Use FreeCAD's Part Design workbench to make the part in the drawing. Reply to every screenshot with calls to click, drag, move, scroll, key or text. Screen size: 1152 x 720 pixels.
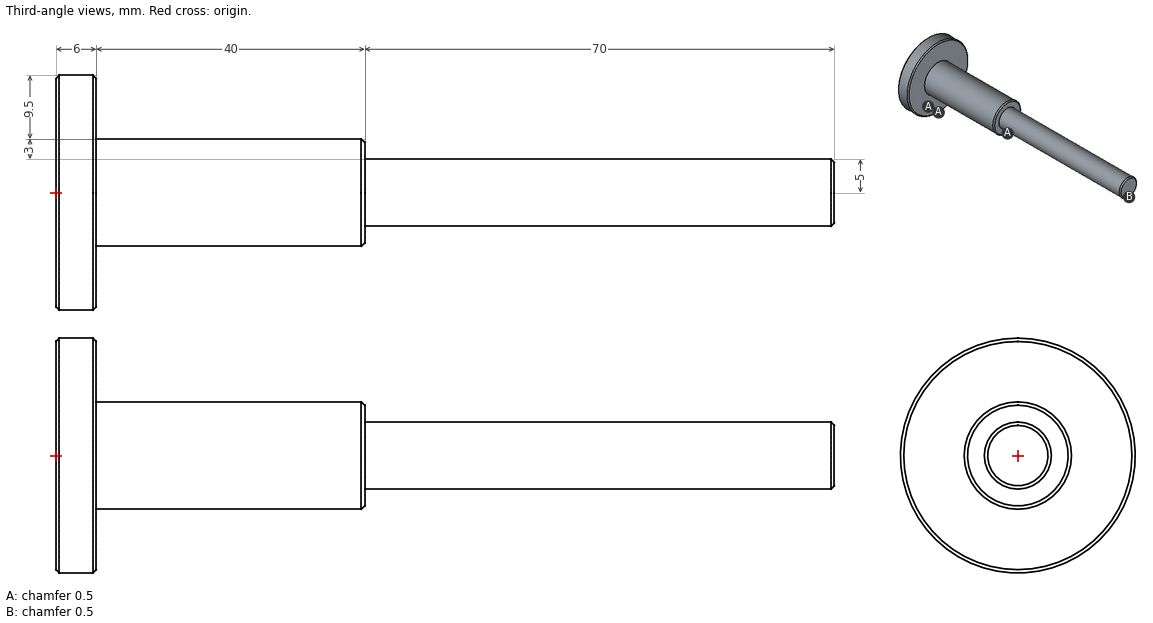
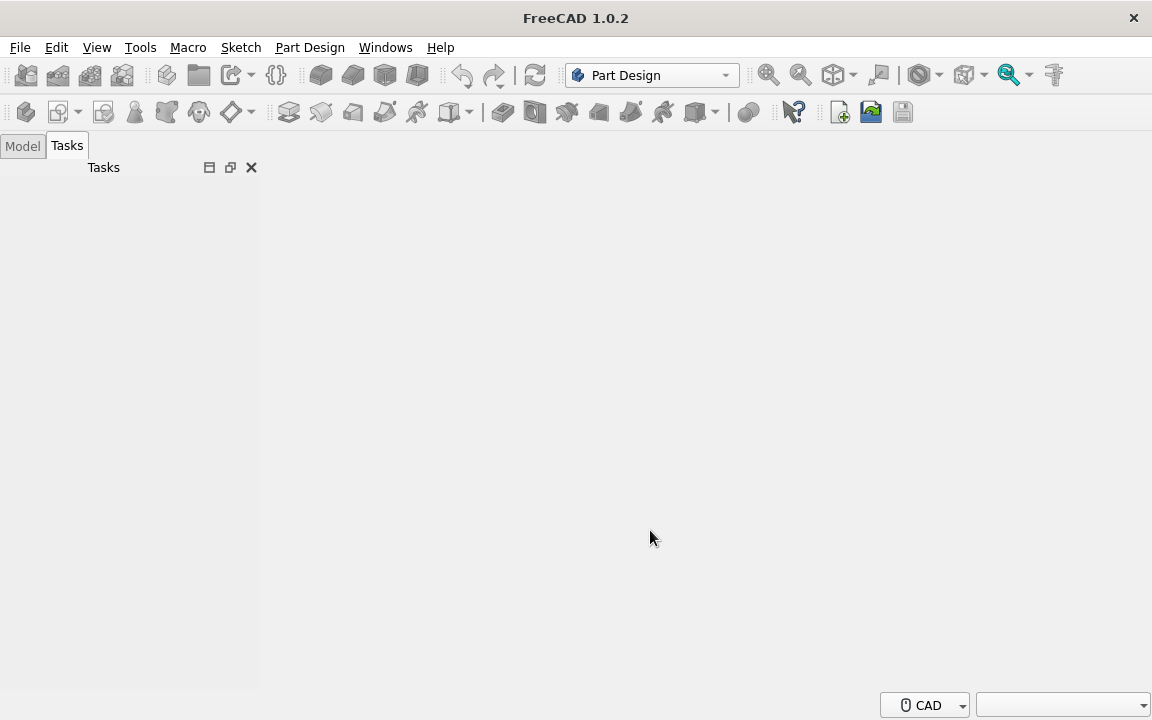
click(840, 112)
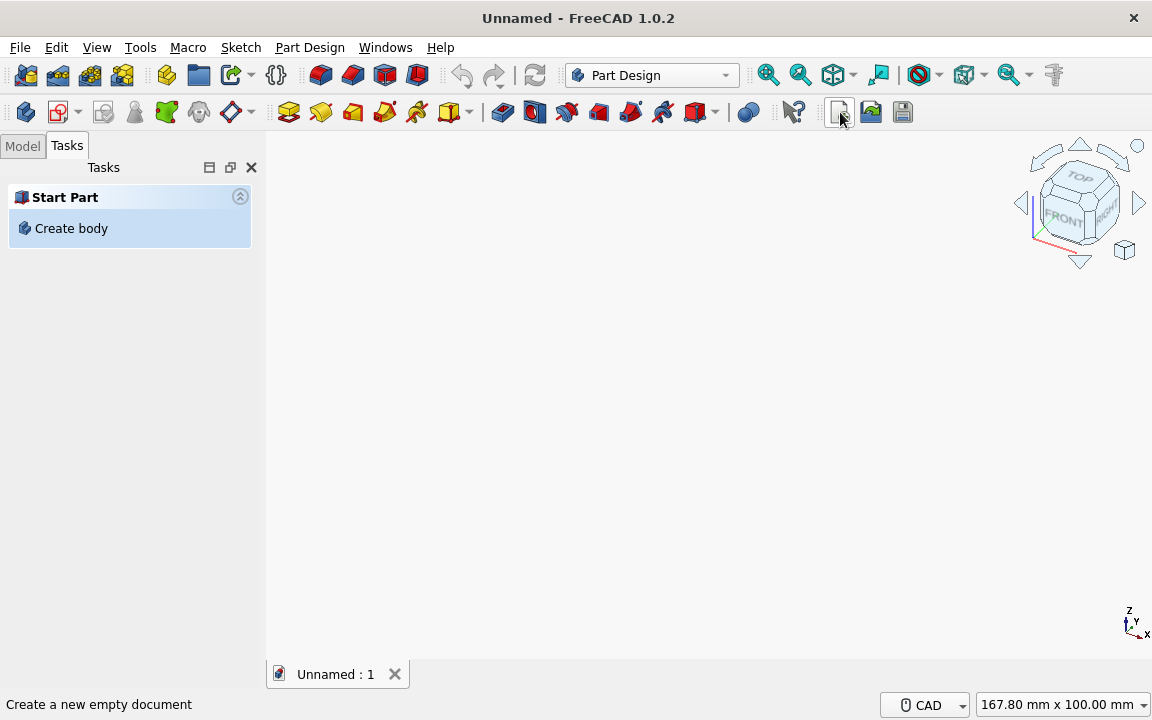
click(58, 112)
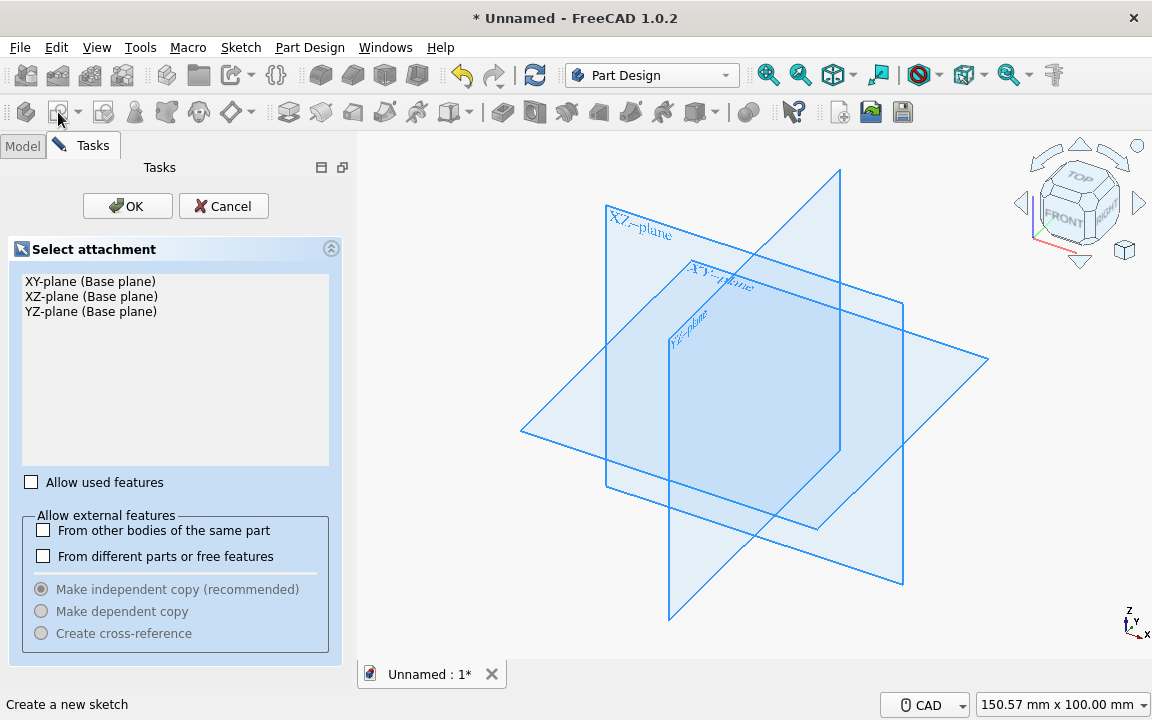
click(82, 282)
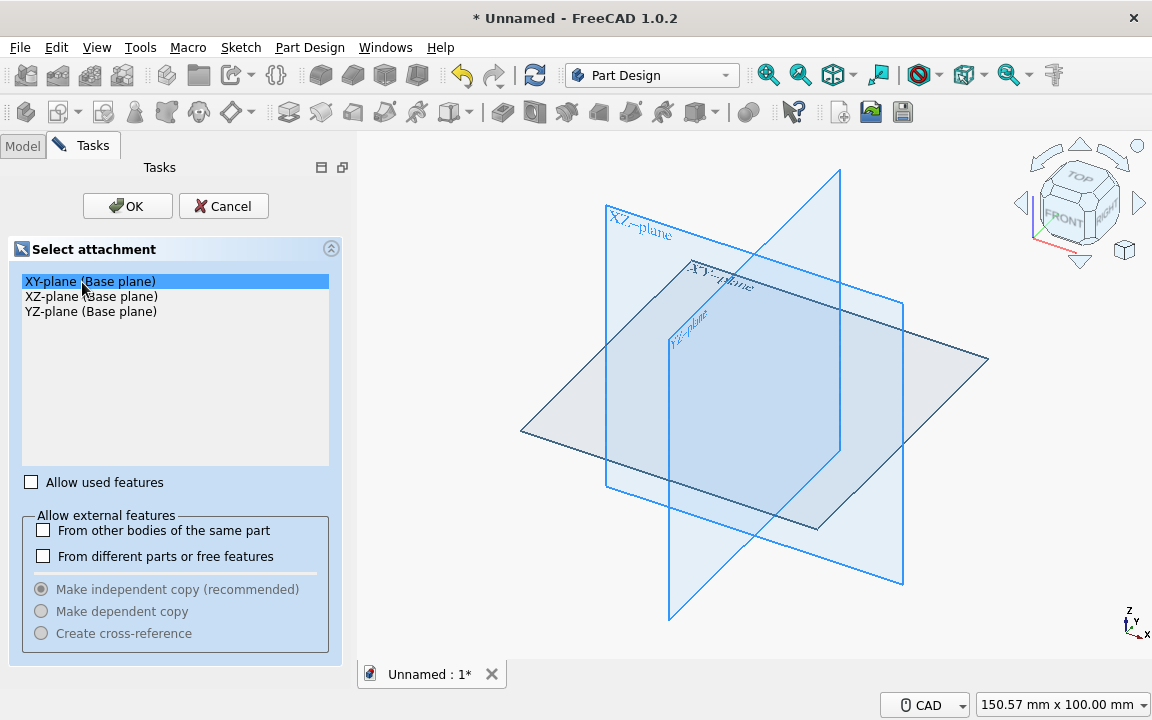
click(128, 206)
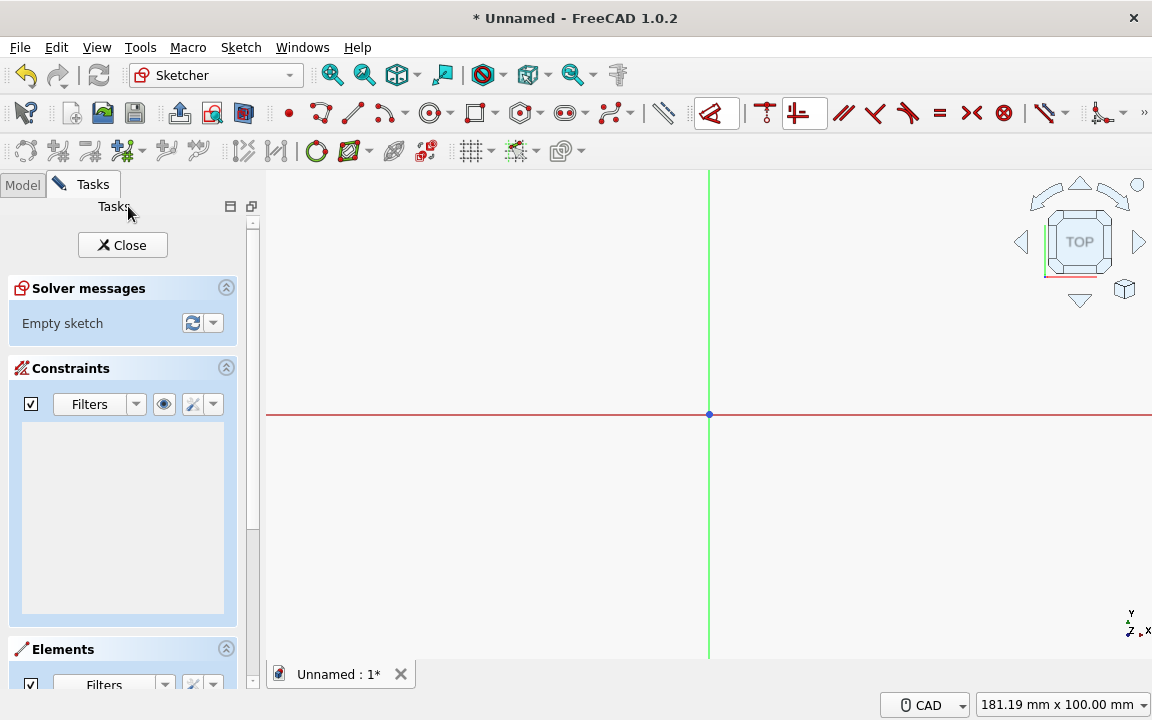
scroll(294, 501, down, 2)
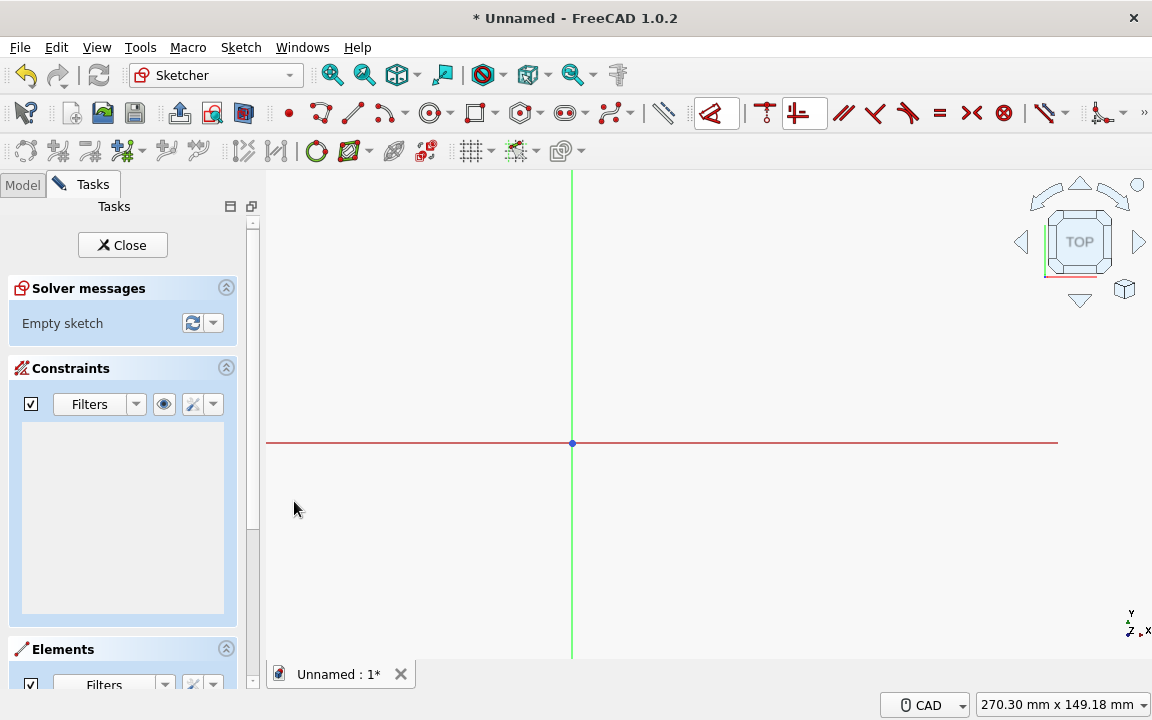
click(322, 114)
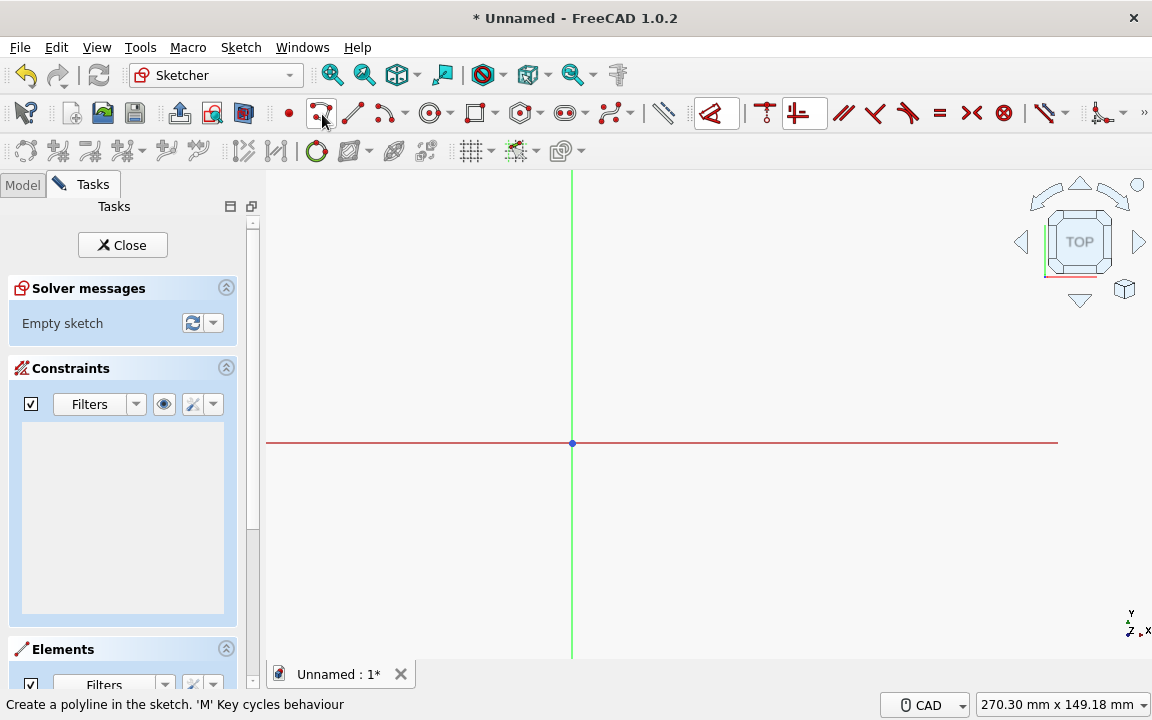
click(572, 443)
click(952, 434)
click(952, 427)
click(723, 427)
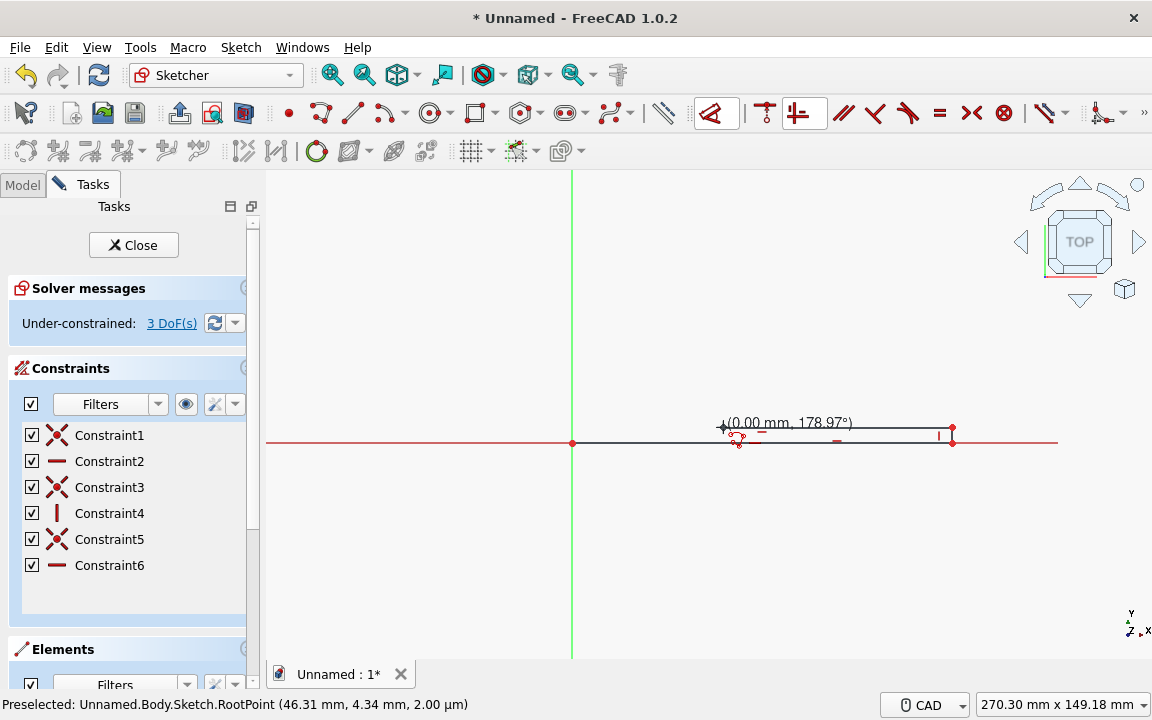
scroll(723, 417, up, 3)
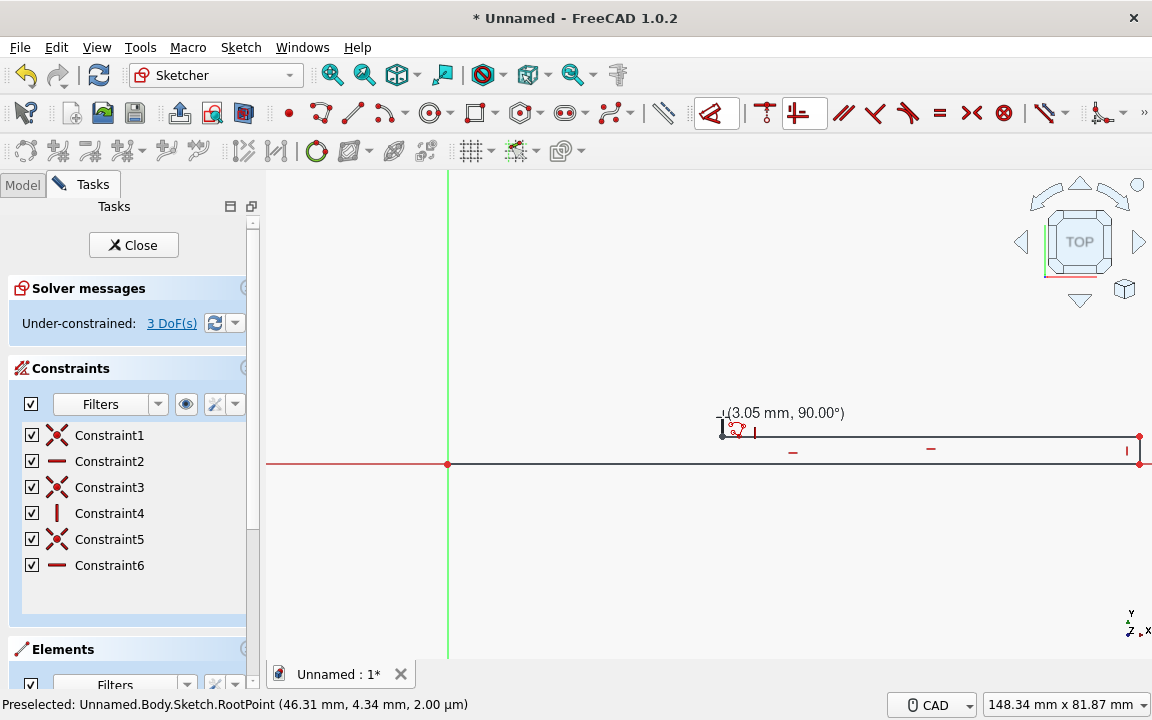
click(723, 417)
click(484, 417)
click(484, 360)
click(457, 360)
click(448, 464)
key(Escape)
key(Escape)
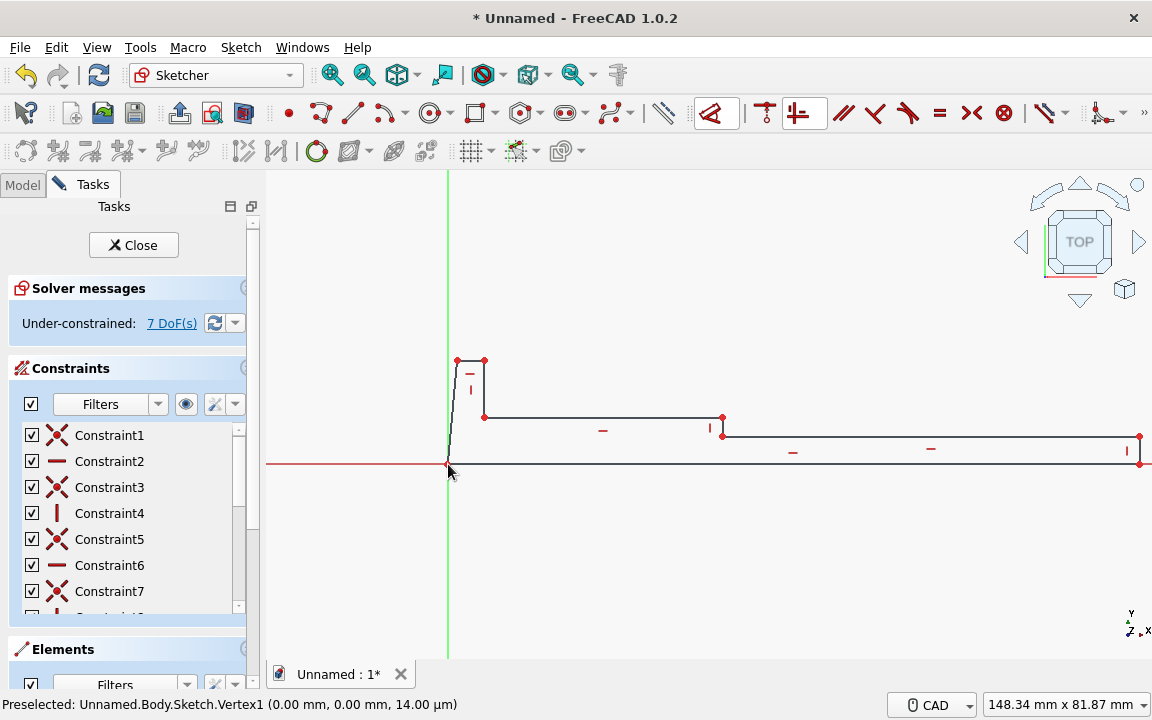
click(451, 433)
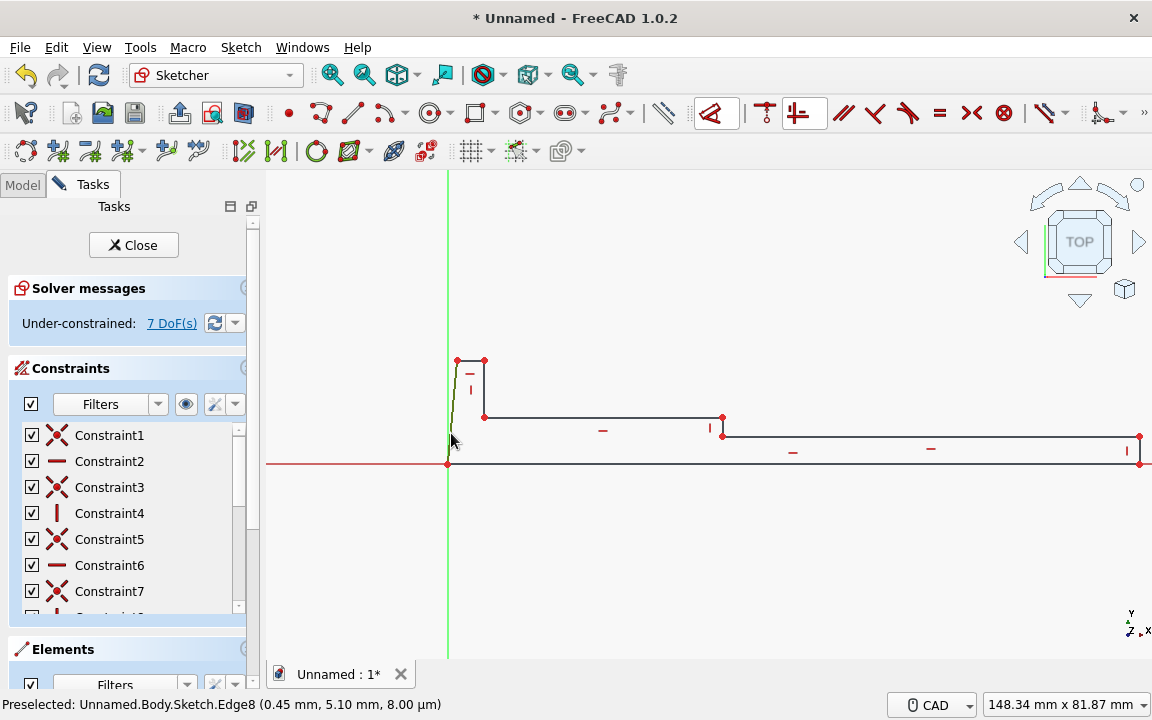
click(822, 114)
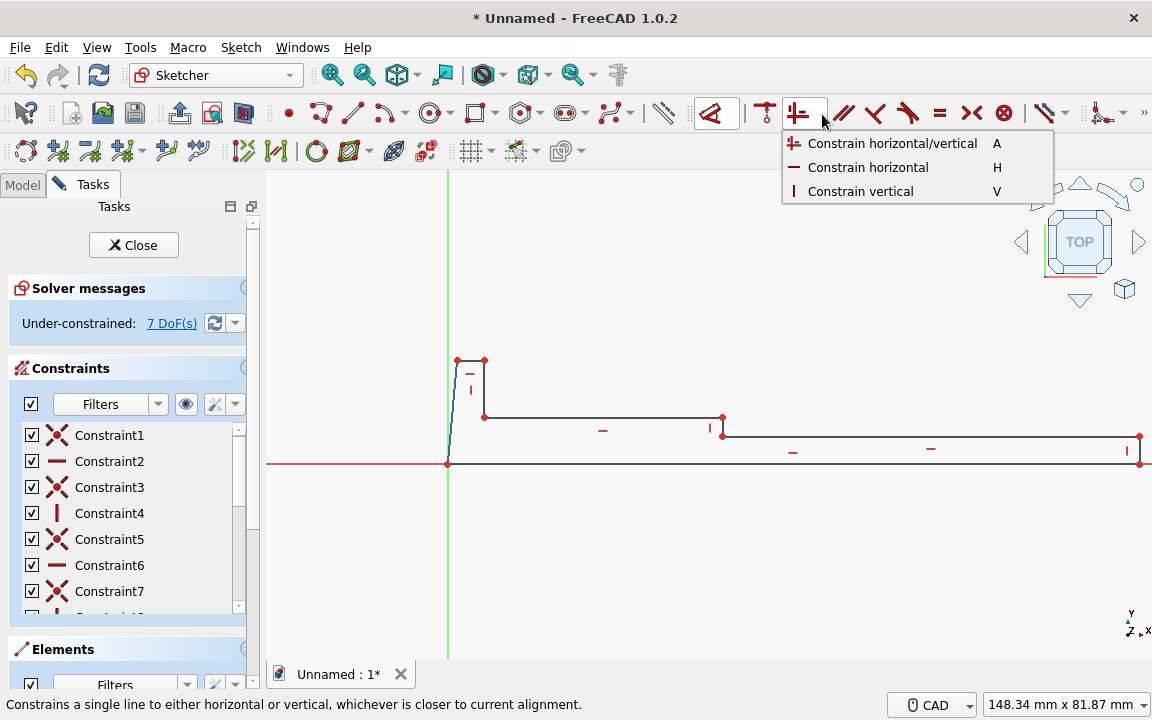
click(918, 191)